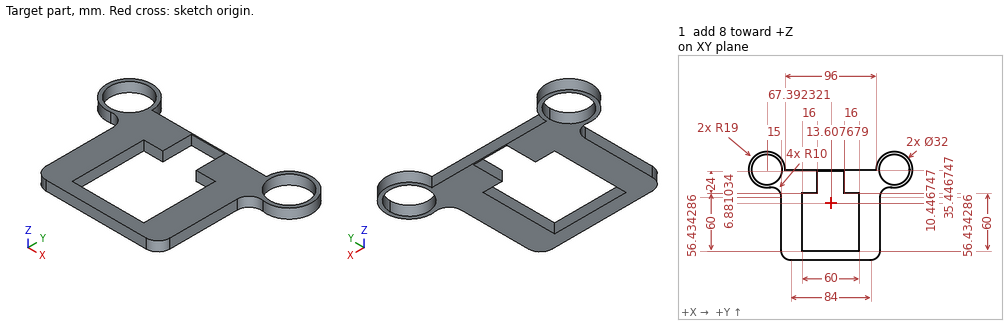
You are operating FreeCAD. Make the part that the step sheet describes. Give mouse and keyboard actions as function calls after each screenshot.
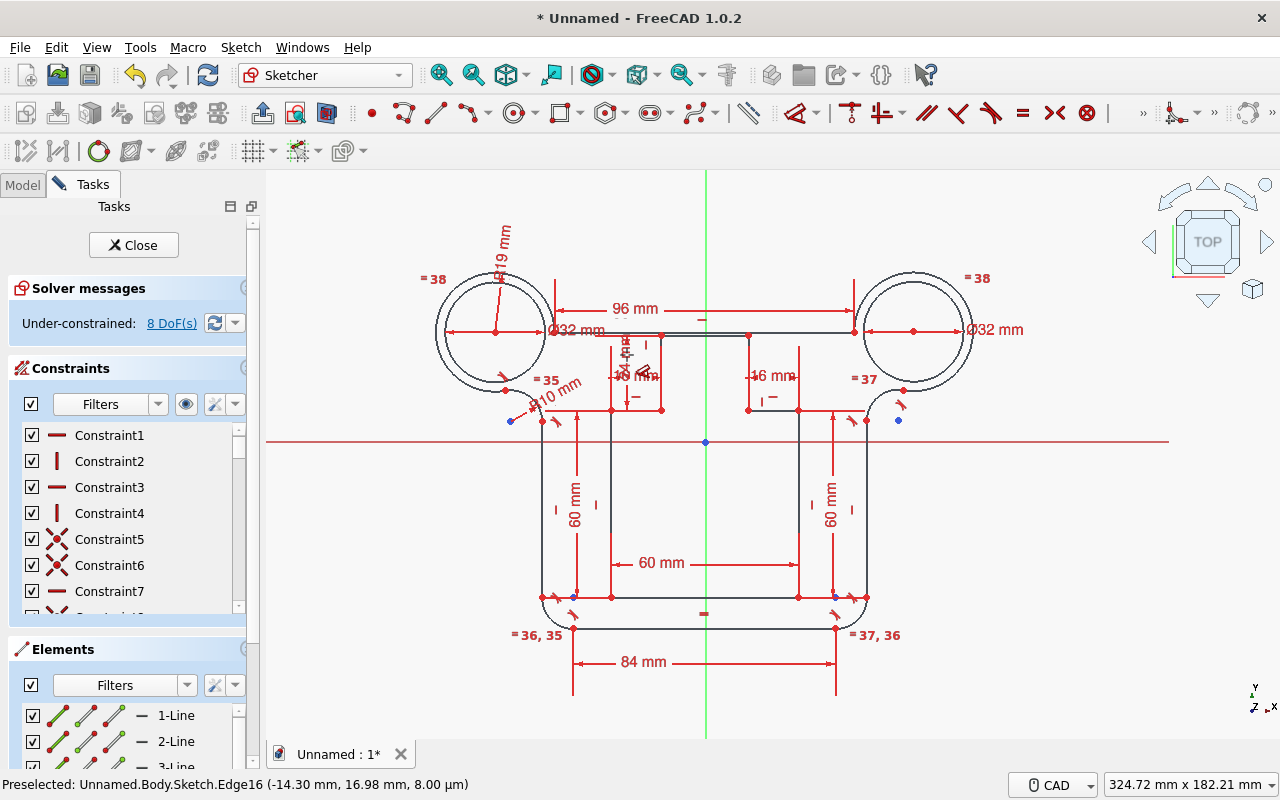
click(542, 422)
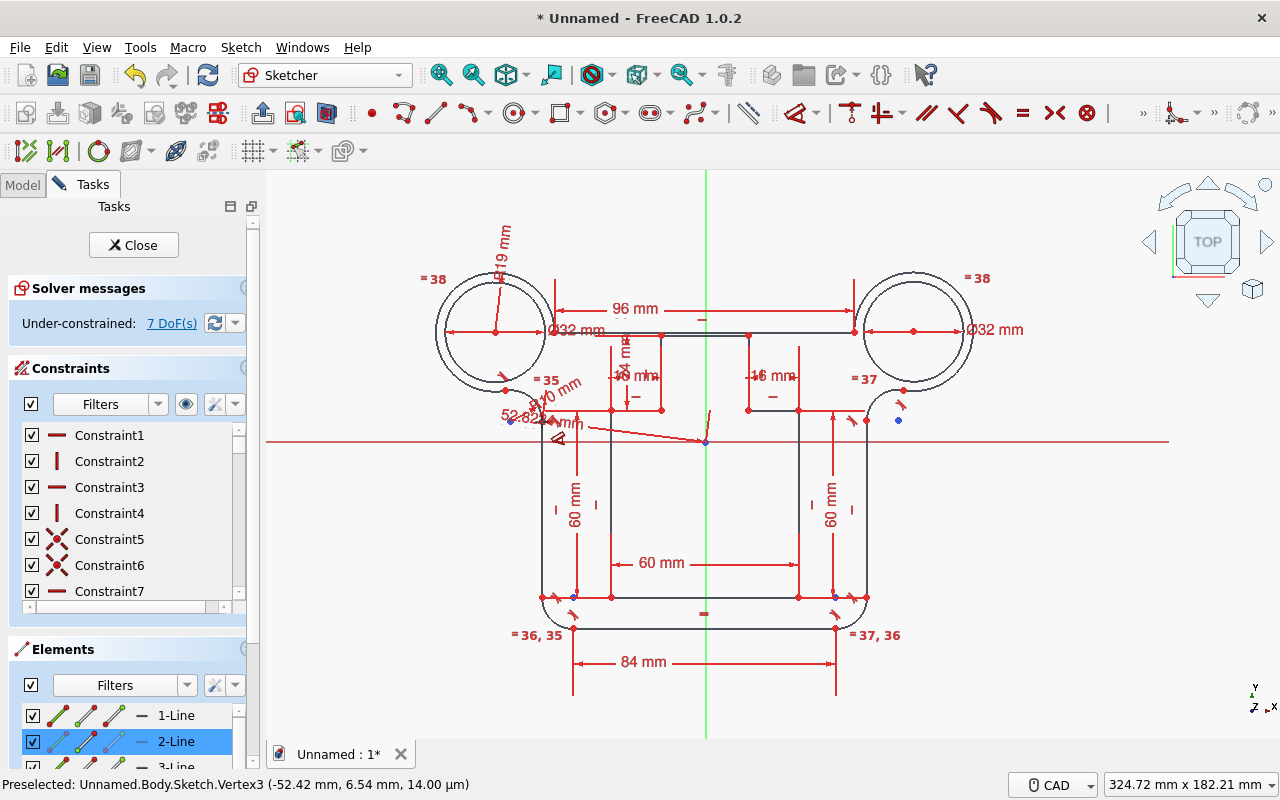
click(495, 332)
click(508, 298)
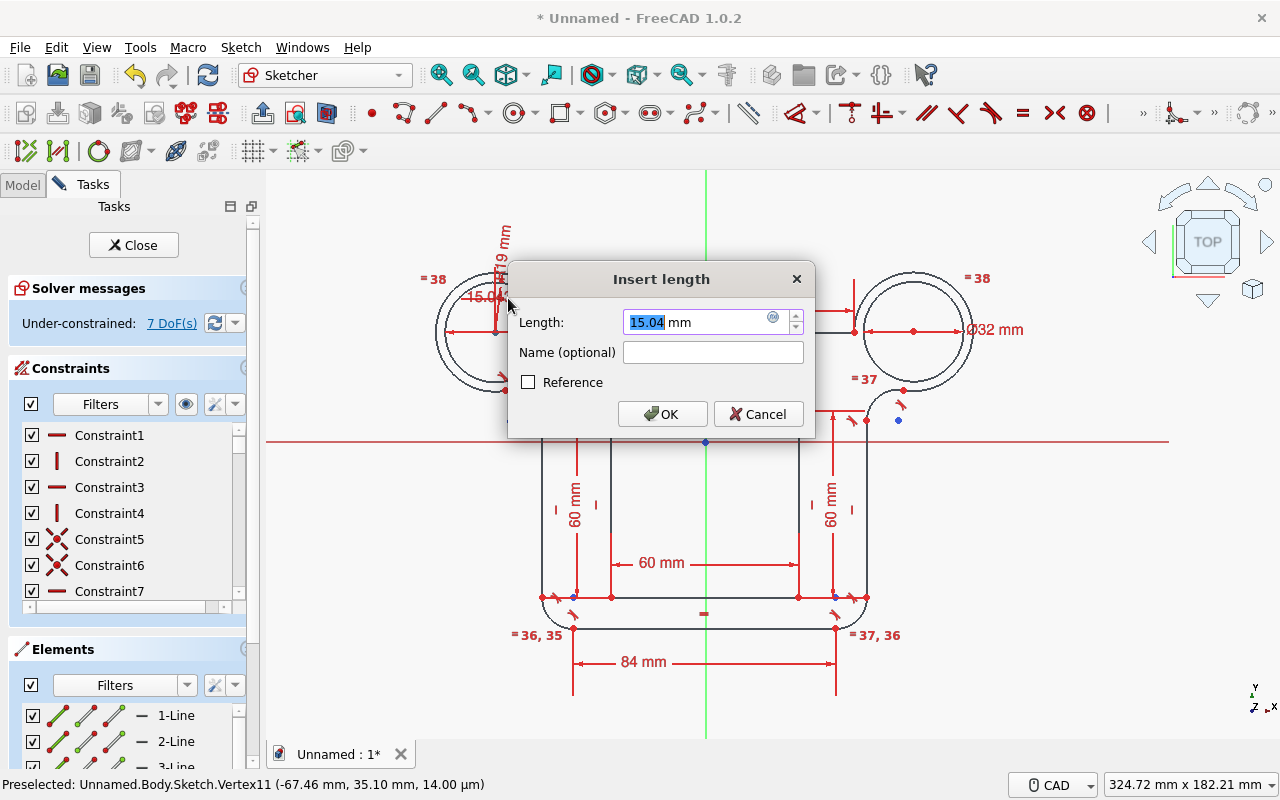
text(15)
key(Return)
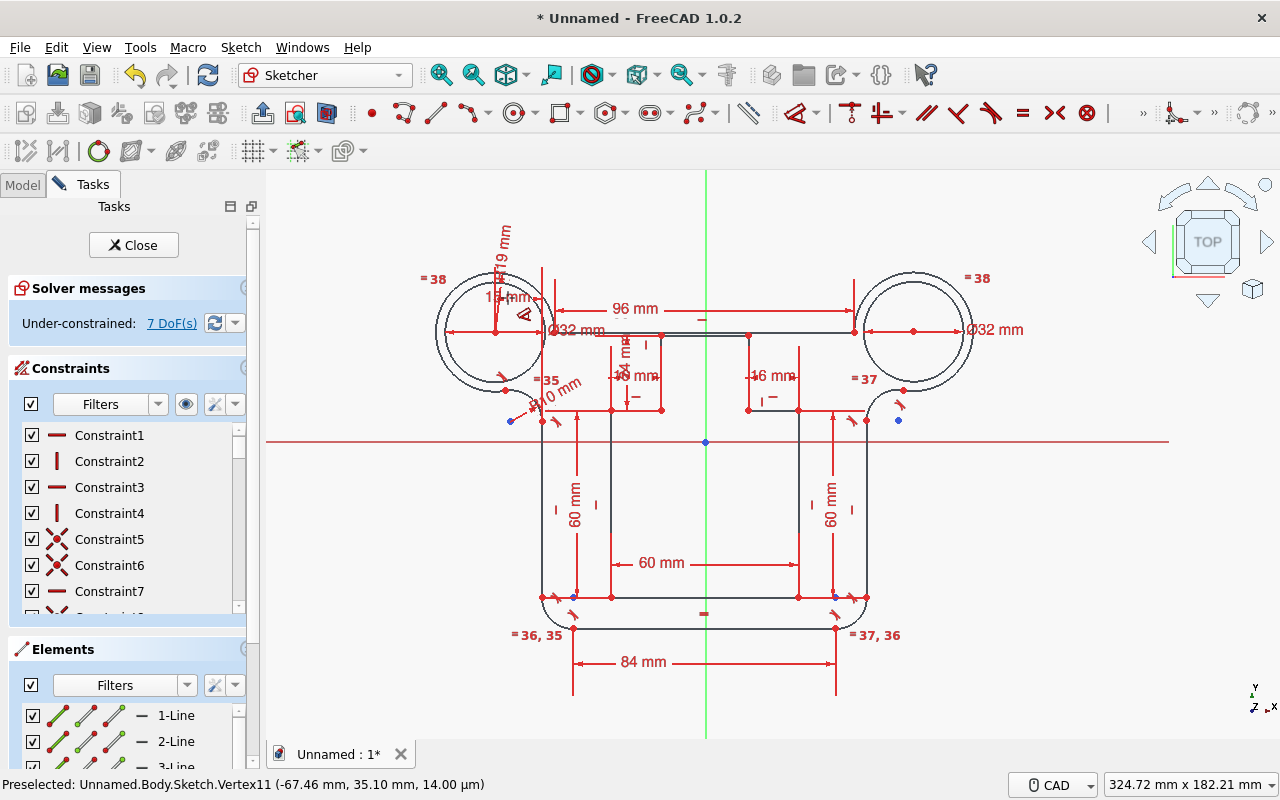
click(542, 474)
click(508, 469)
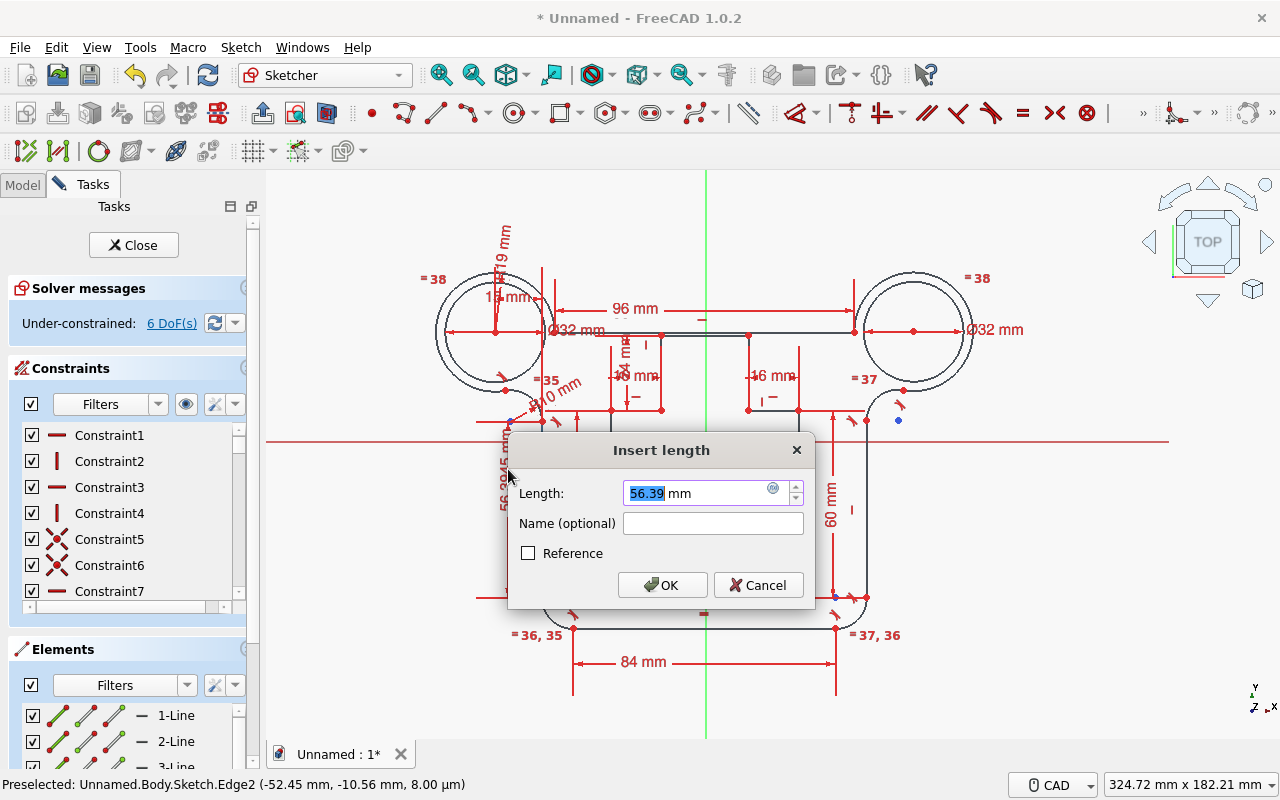
text(56.434286)
key(Return)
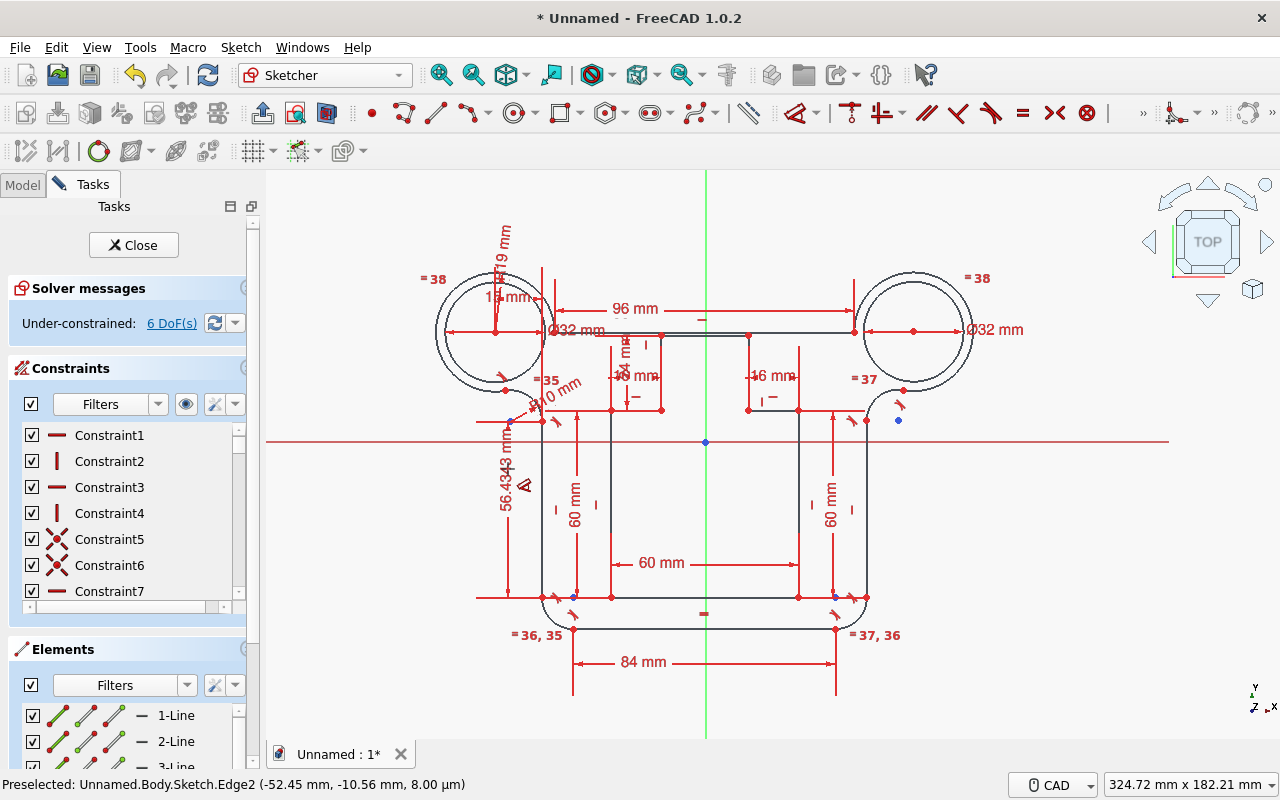
click(867, 545)
click(901, 469)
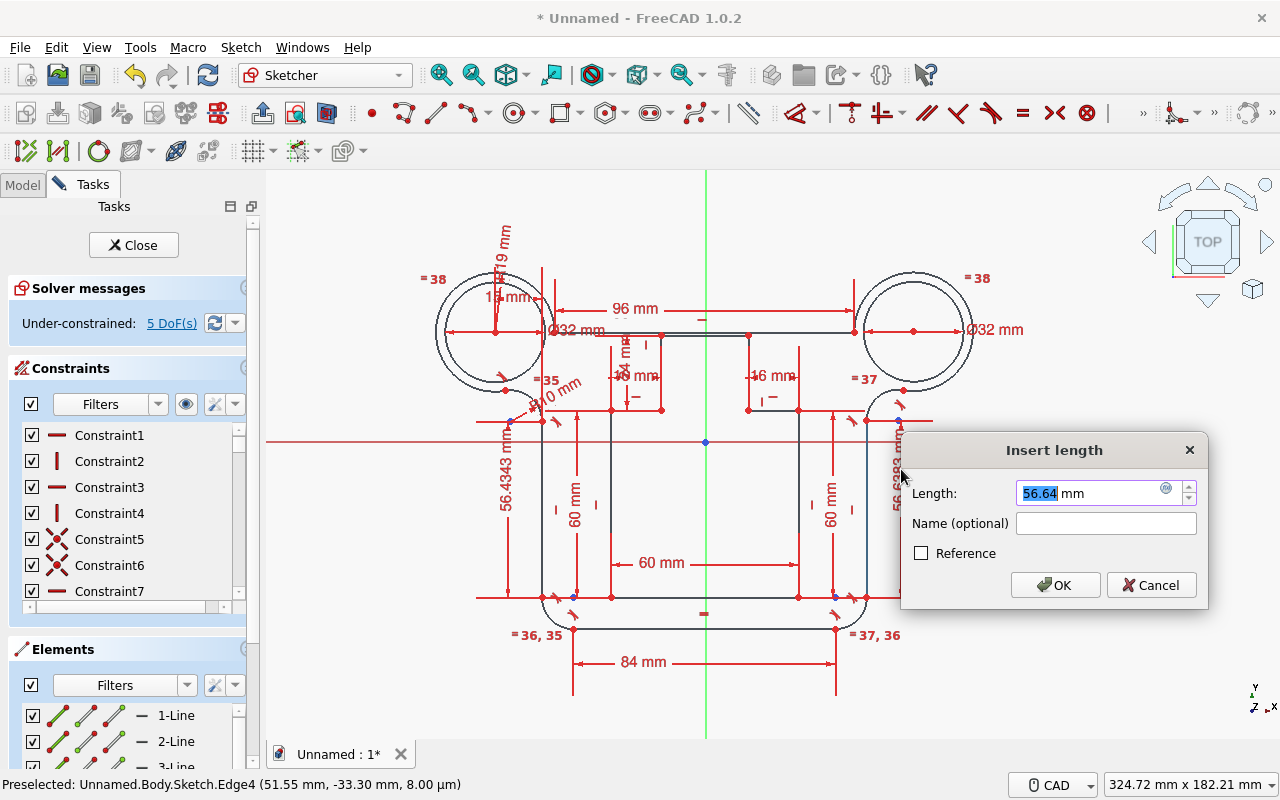
text(56.434286)
key(Return)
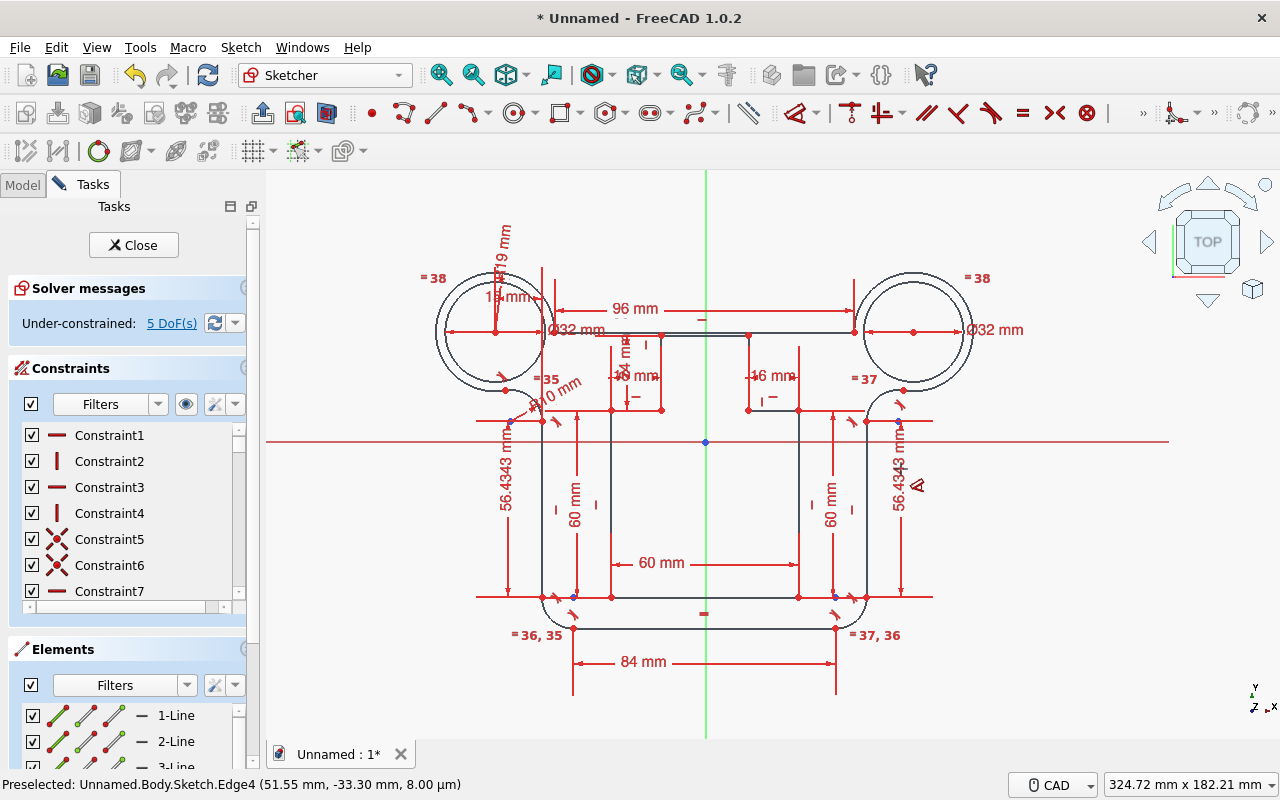
scroll(542, 421, up, 4)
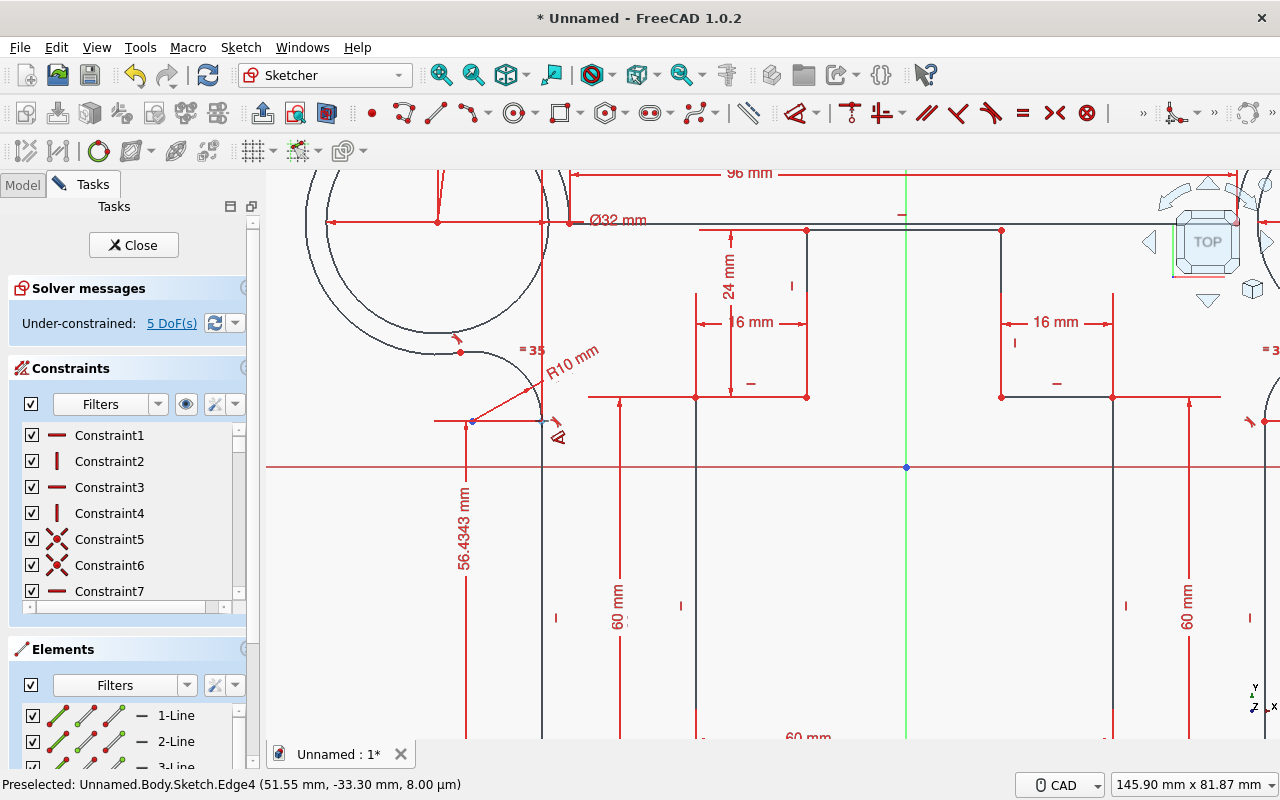
click(542, 421)
click(508, 444)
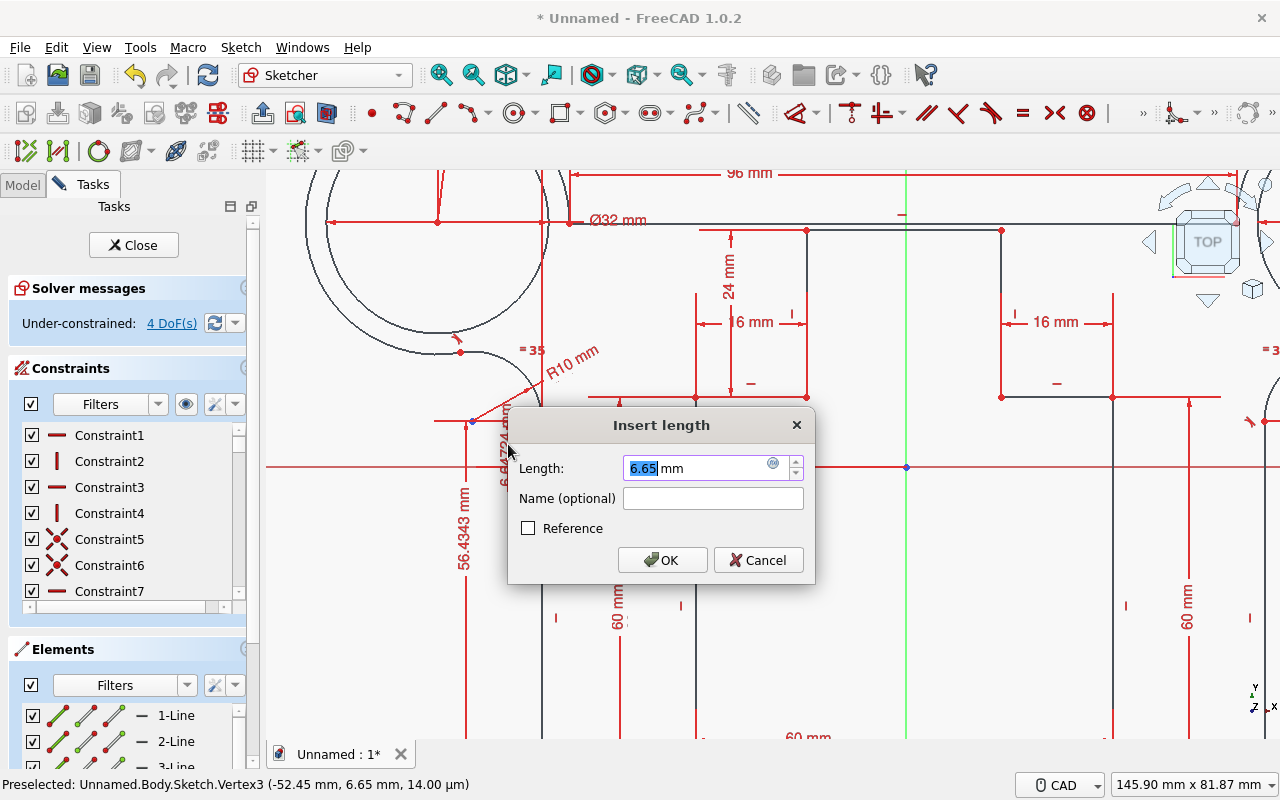
text(6.881034)
key(Return)